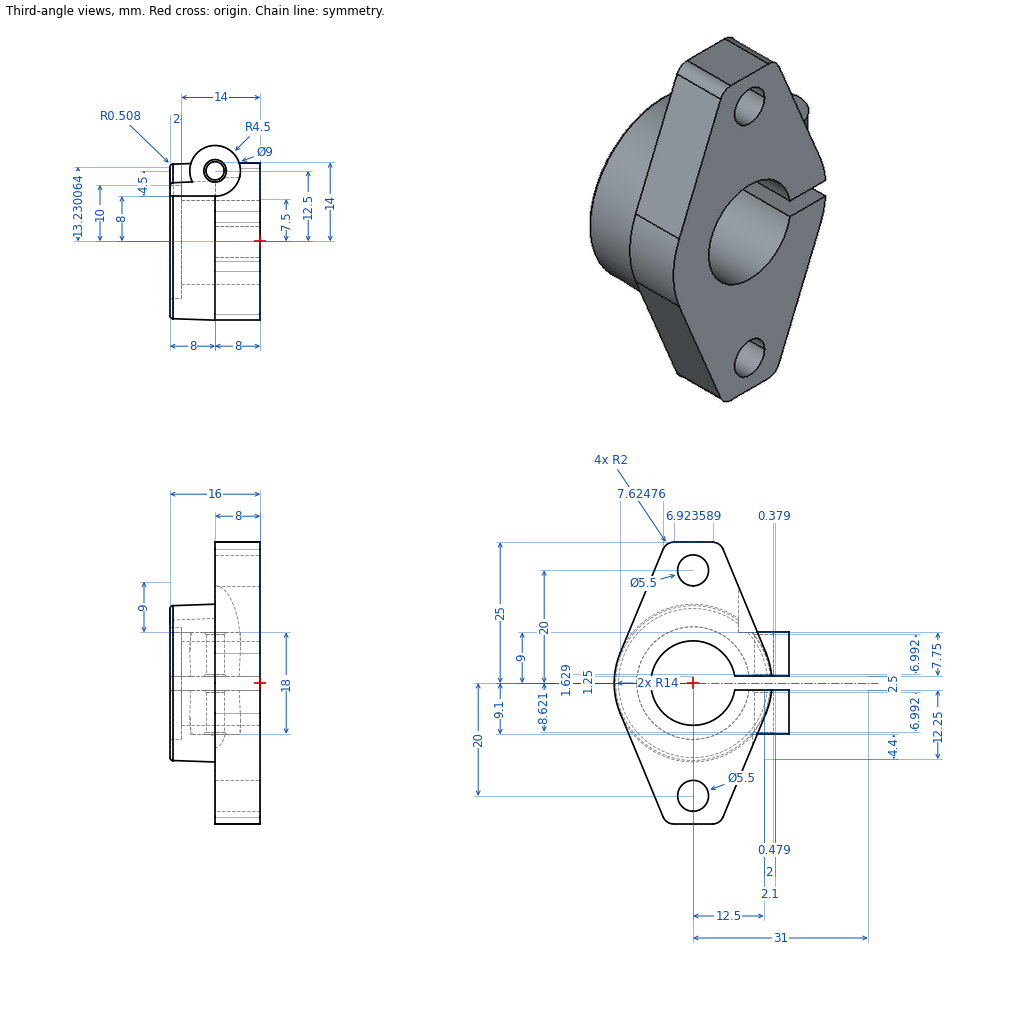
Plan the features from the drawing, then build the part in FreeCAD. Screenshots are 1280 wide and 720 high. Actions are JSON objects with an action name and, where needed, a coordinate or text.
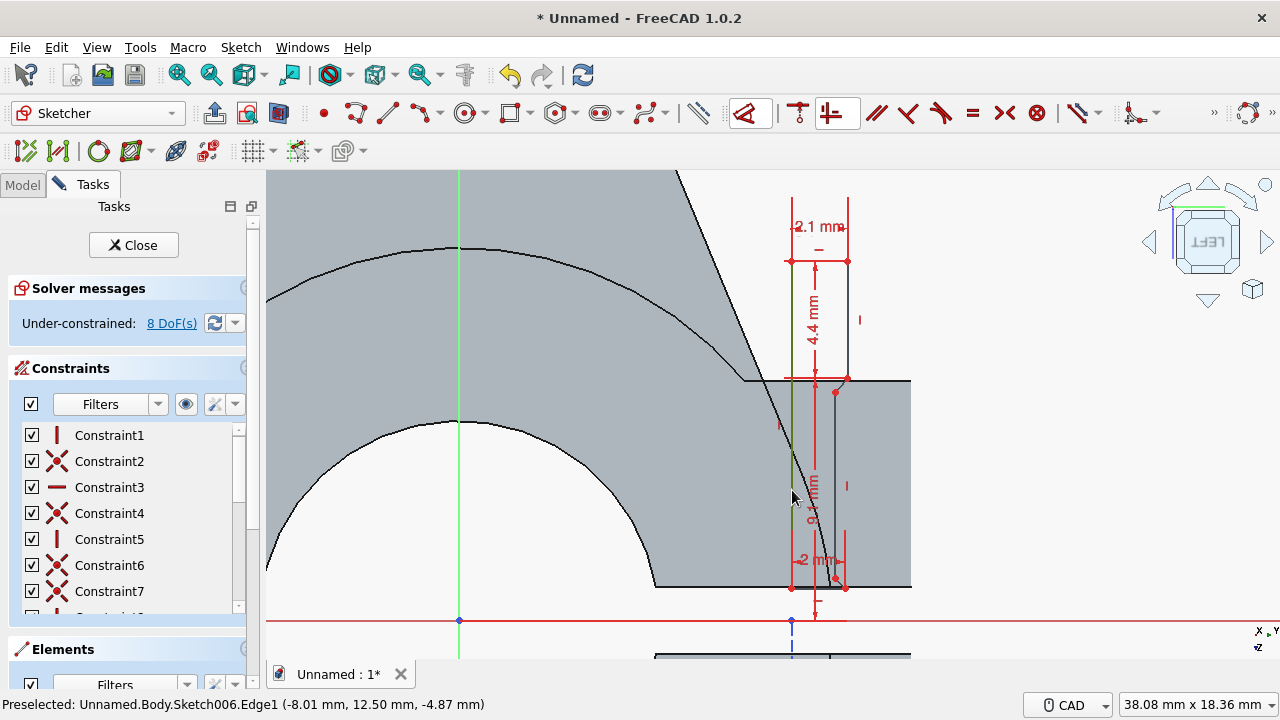
{"action": "left_click", "coordinate": [766, 114]}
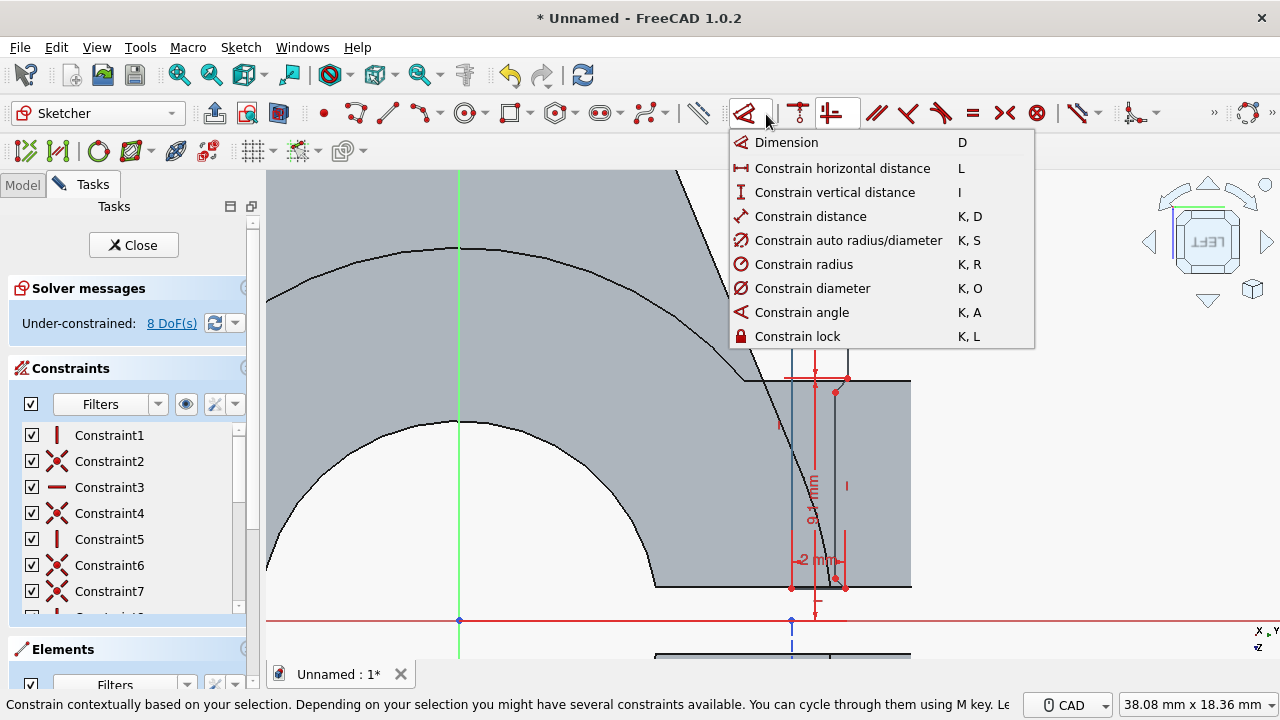
{"action": "left_click", "coordinate": [882, 192]}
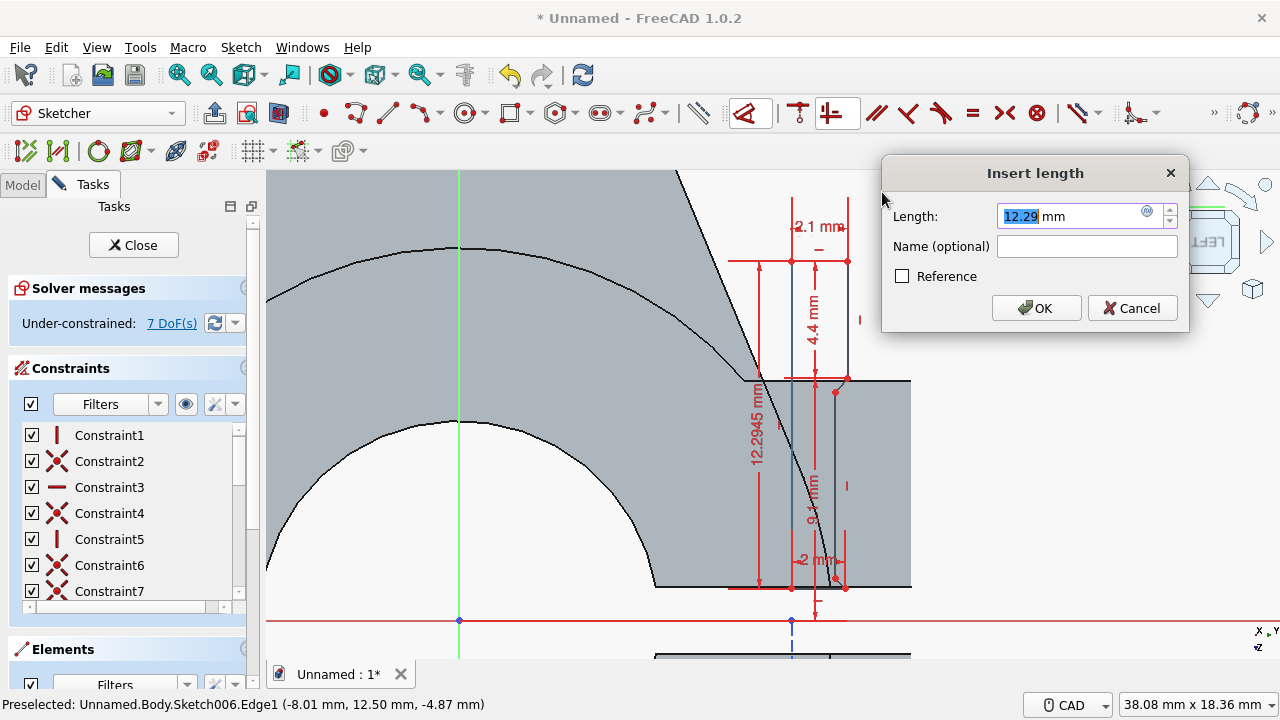
{"action": "type", "text": "12.25"}
{"action": "key", "text": "Return"}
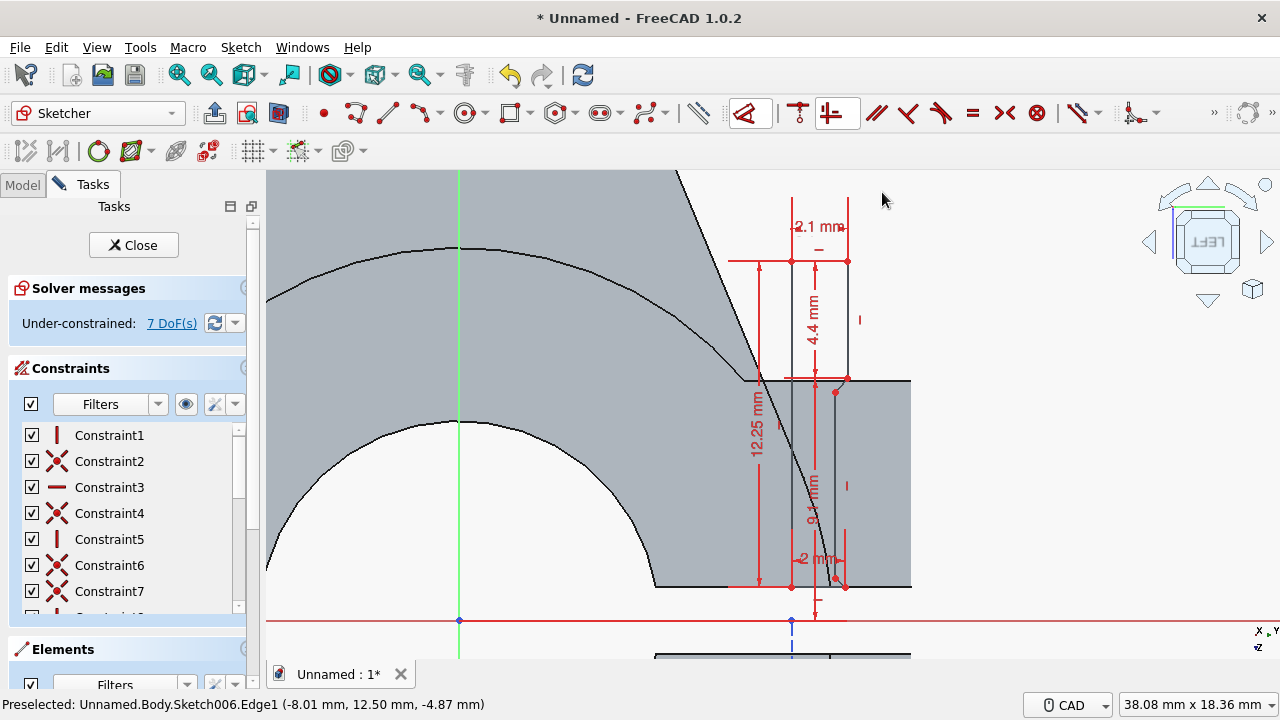
{"action": "left_click", "coordinate": [835, 448]}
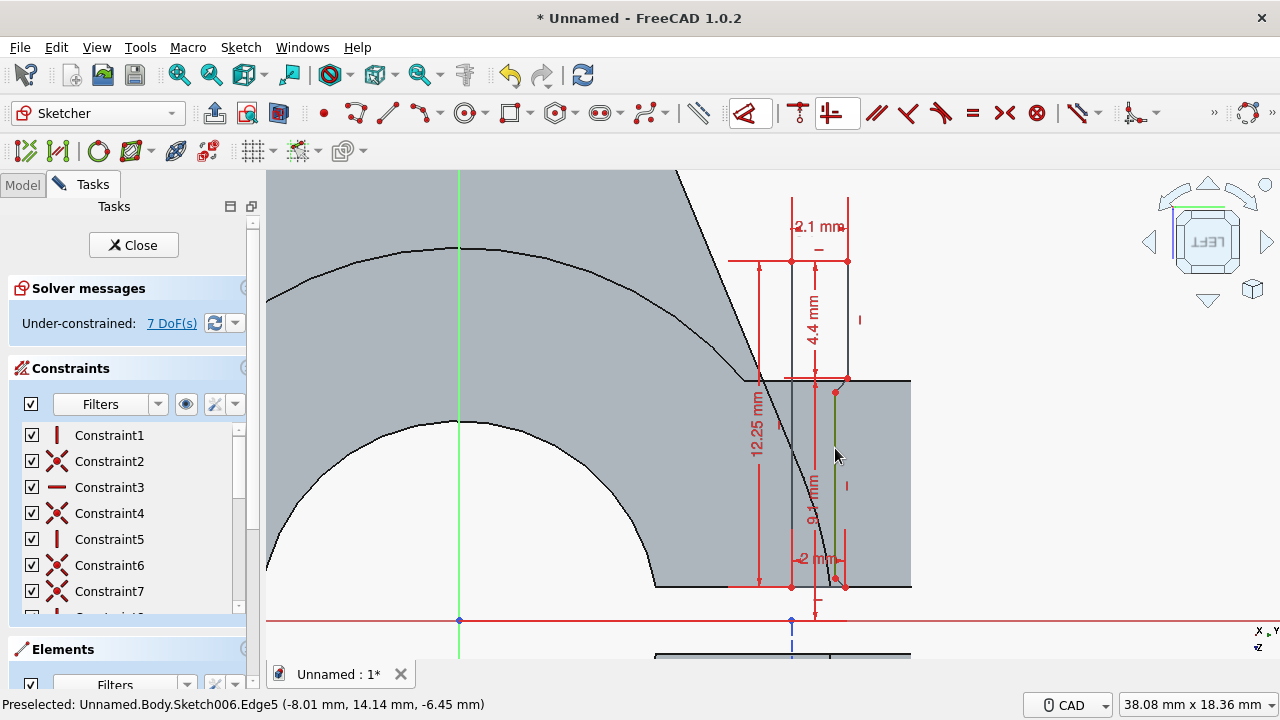
{"action": "key", "text": "i"}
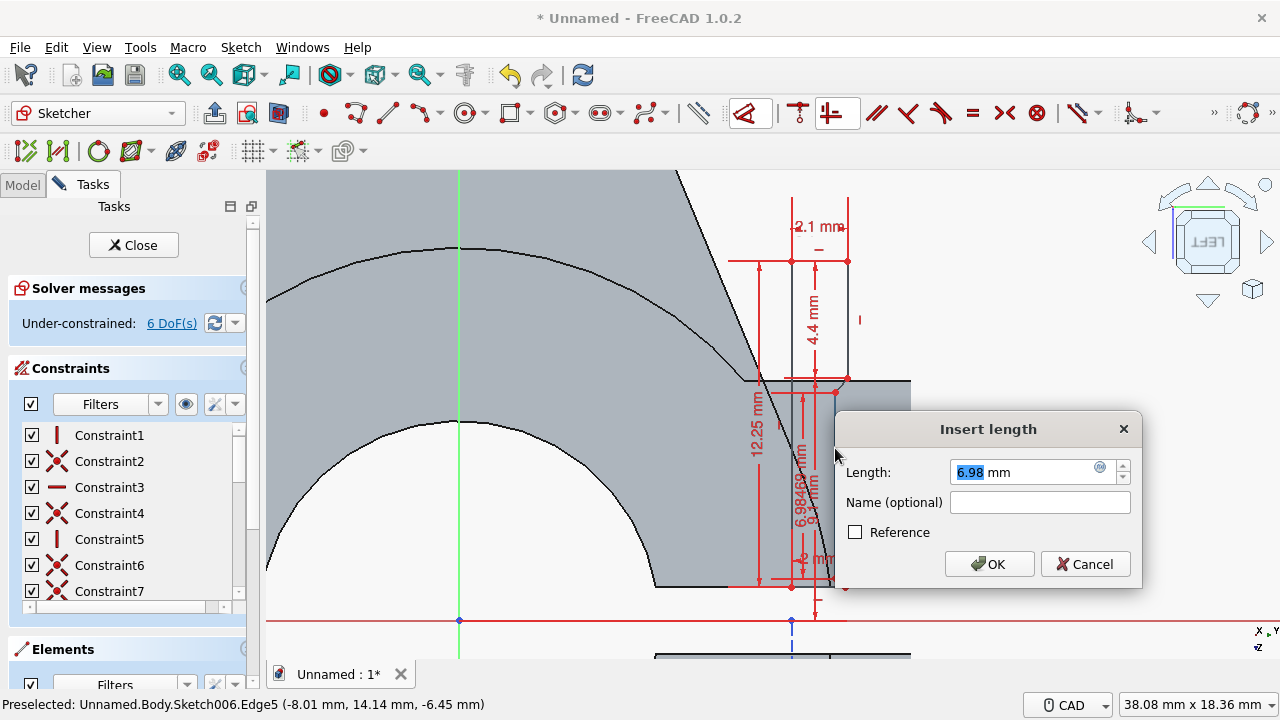
{"action": "type", "text": "6.992"}
{"action": "key", "text": "Return"}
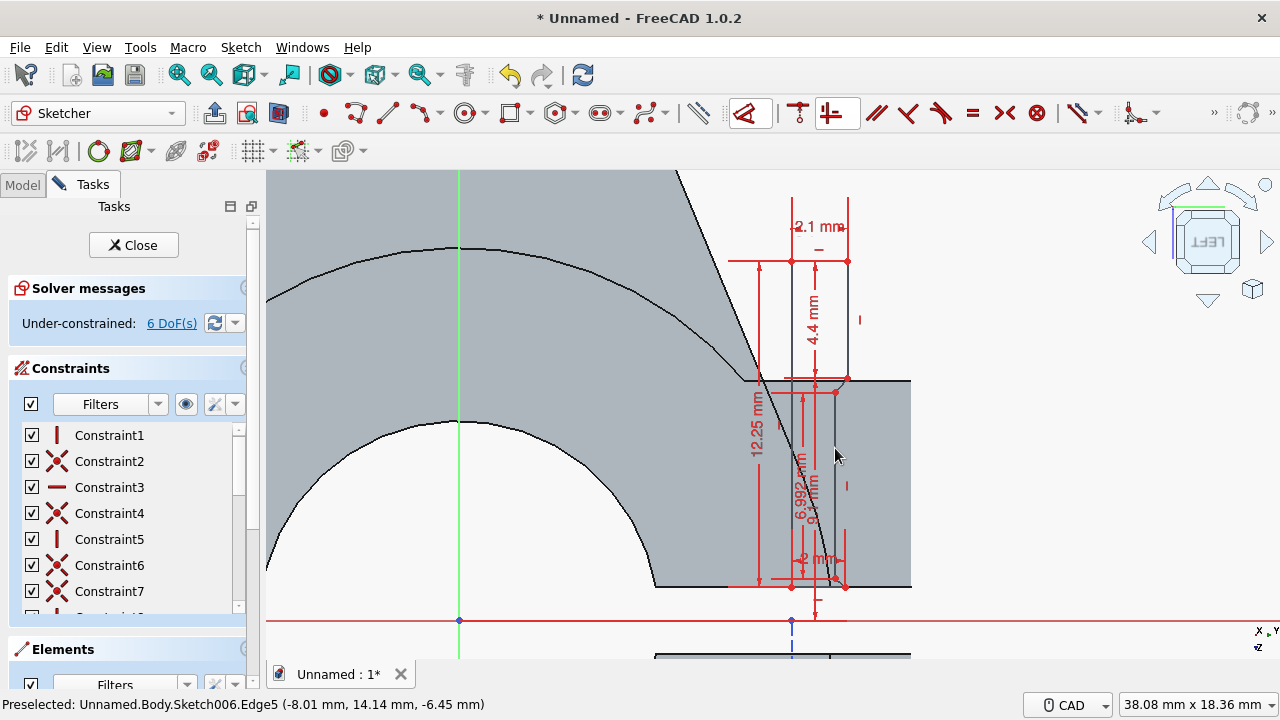
{"action": "left_click", "coordinate": [792, 587]}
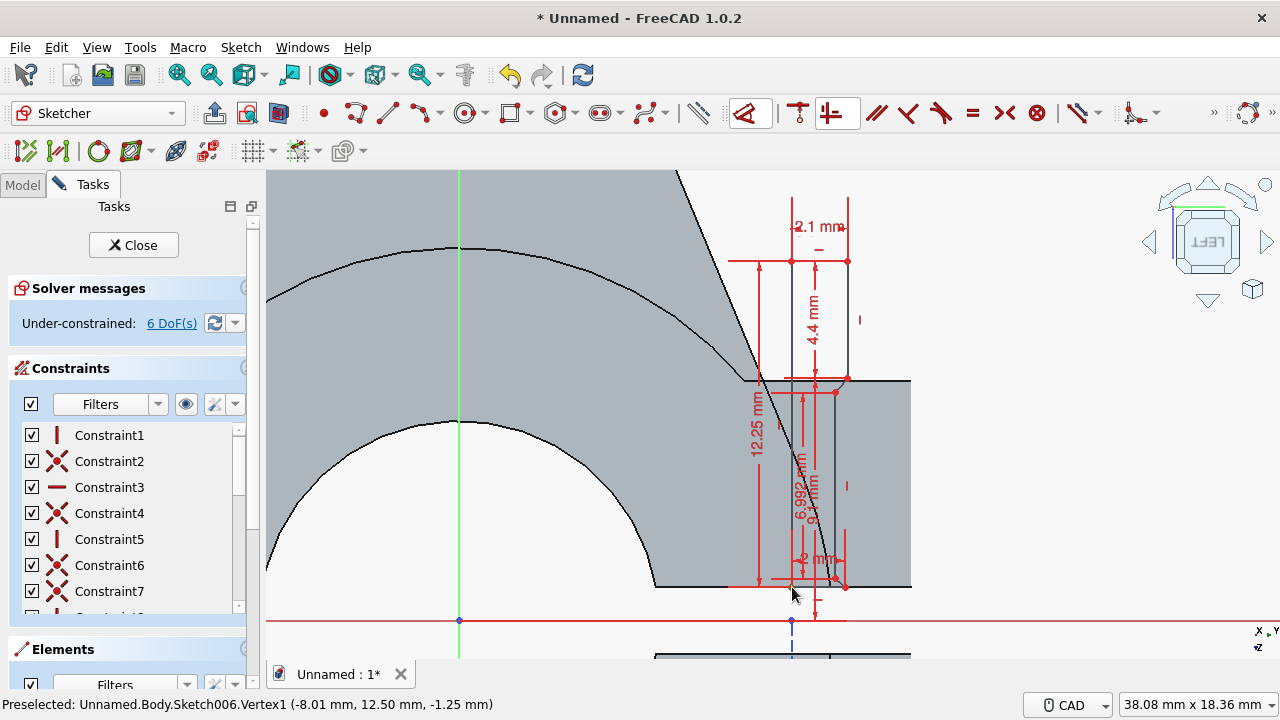
{"action": "key", "text": "l"}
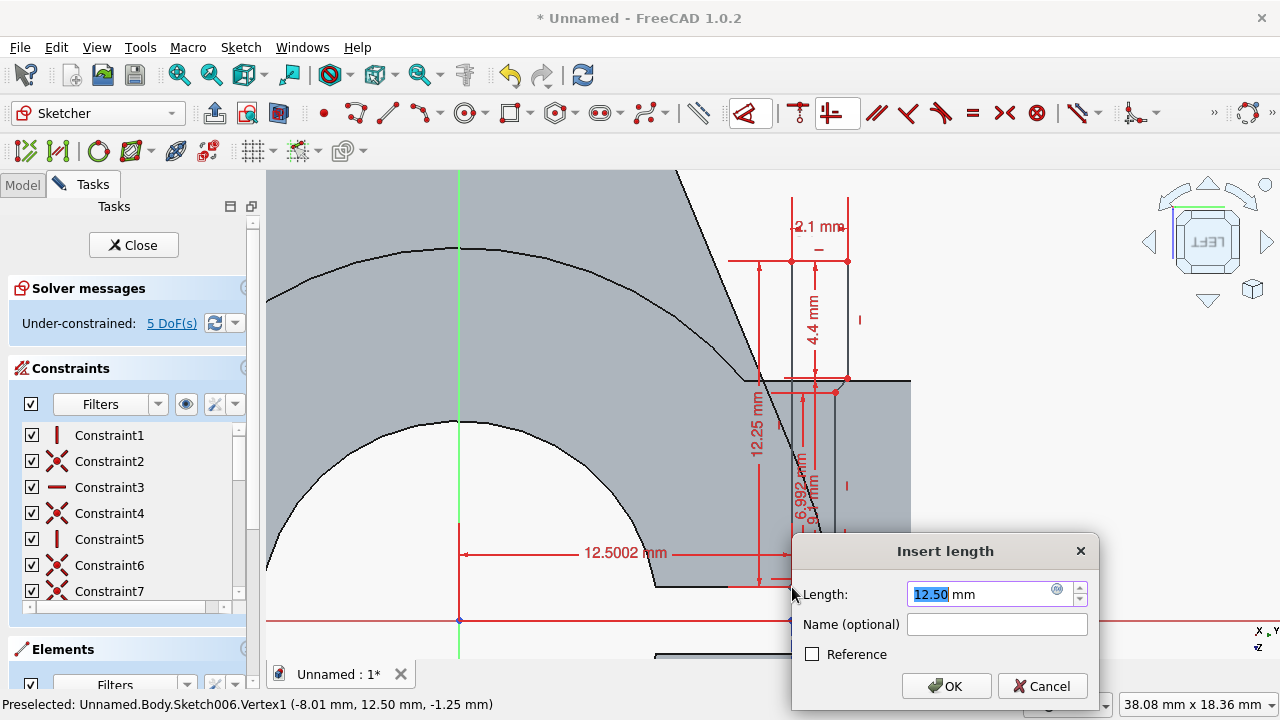
{"action": "type", "text": "12.5"}
{"action": "key", "text": "Return"}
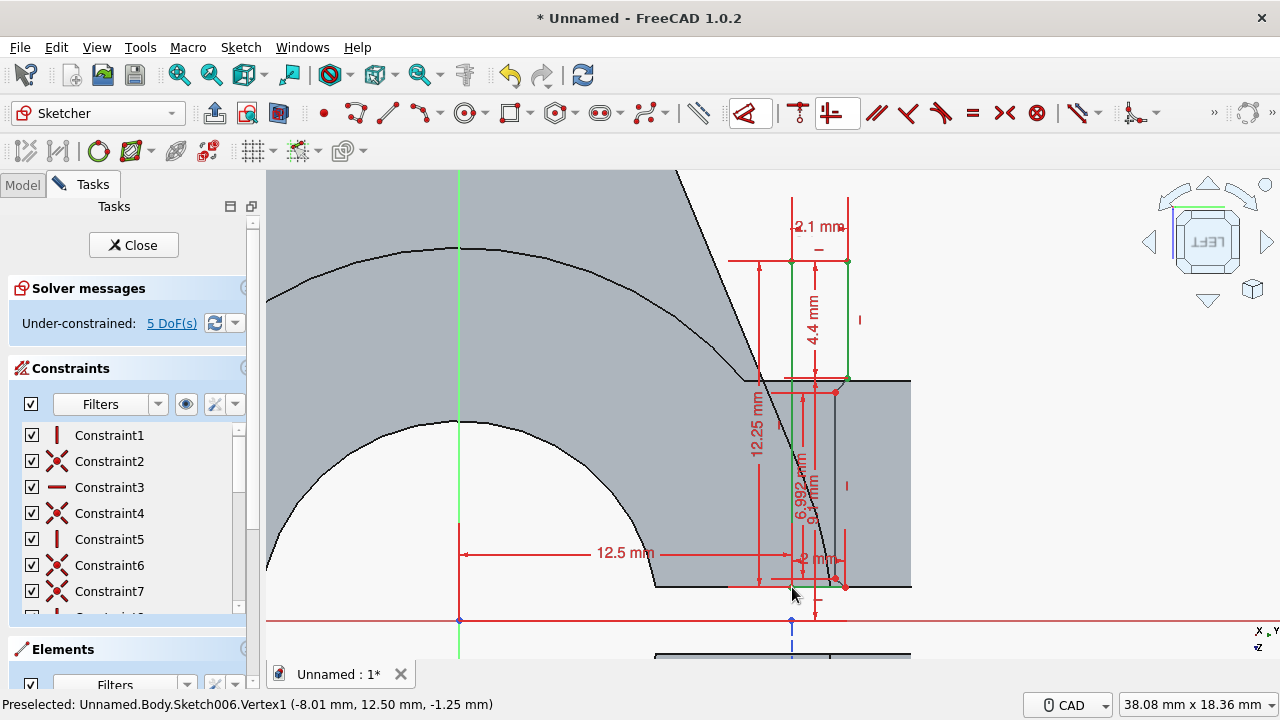
{"action": "left_click", "coordinate": [792, 620]}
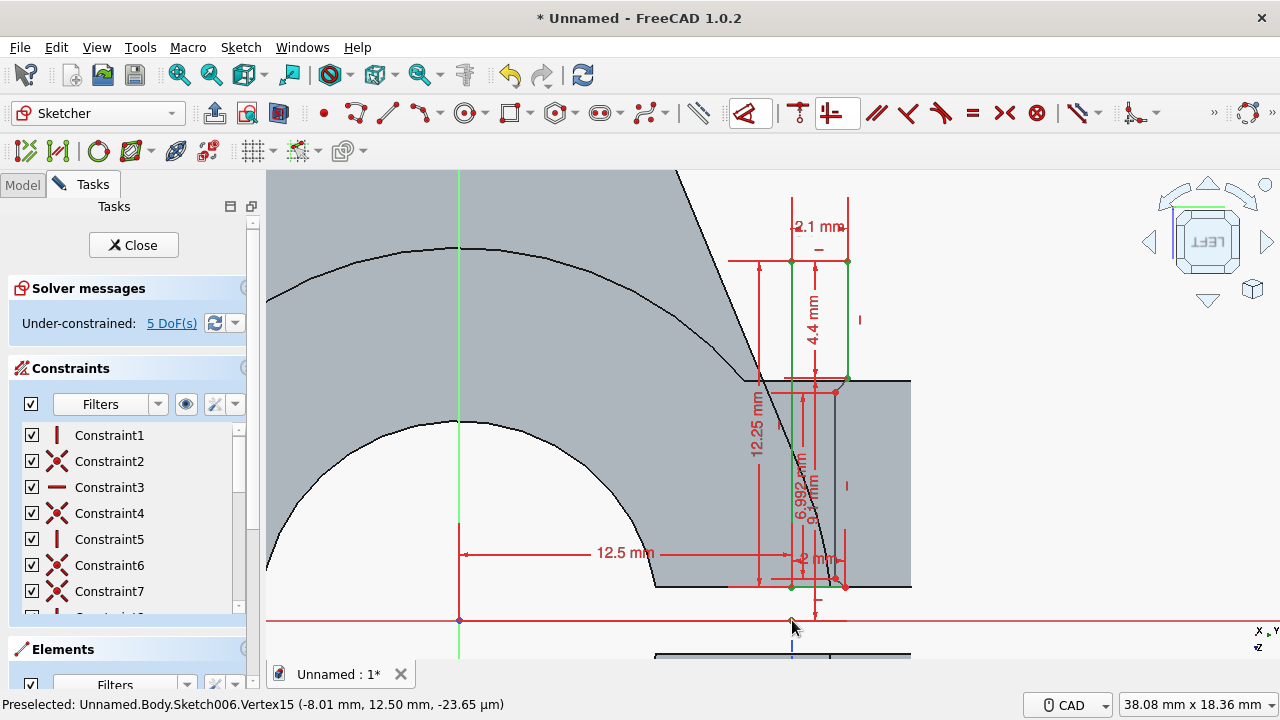
{"action": "left_click", "coordinate": [766, 114]}